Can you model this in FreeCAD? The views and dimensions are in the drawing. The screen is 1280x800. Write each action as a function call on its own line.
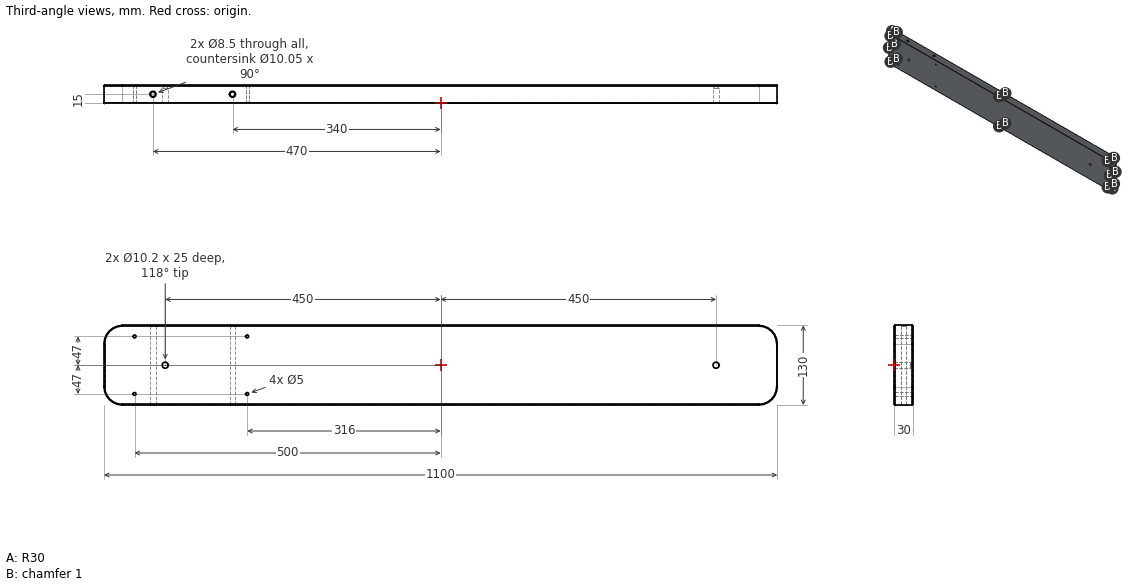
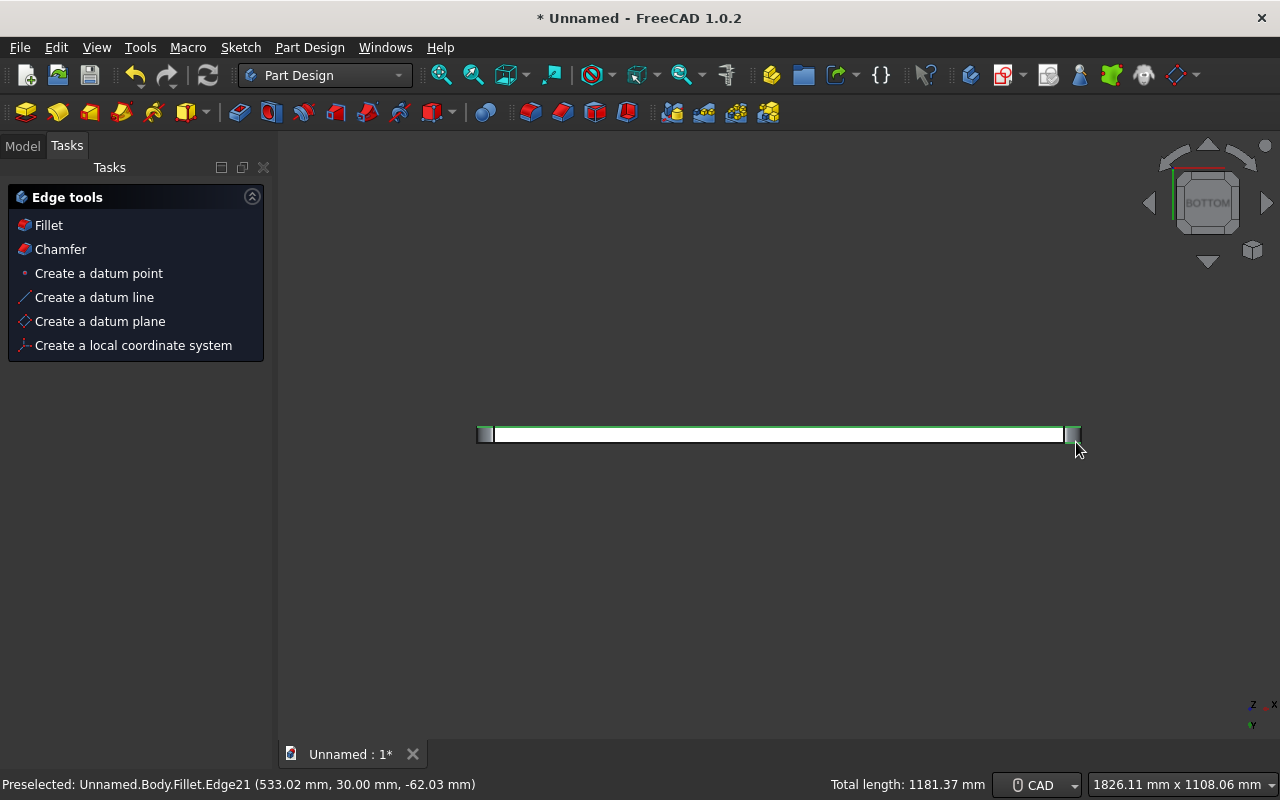
click(482, 442, ctrl)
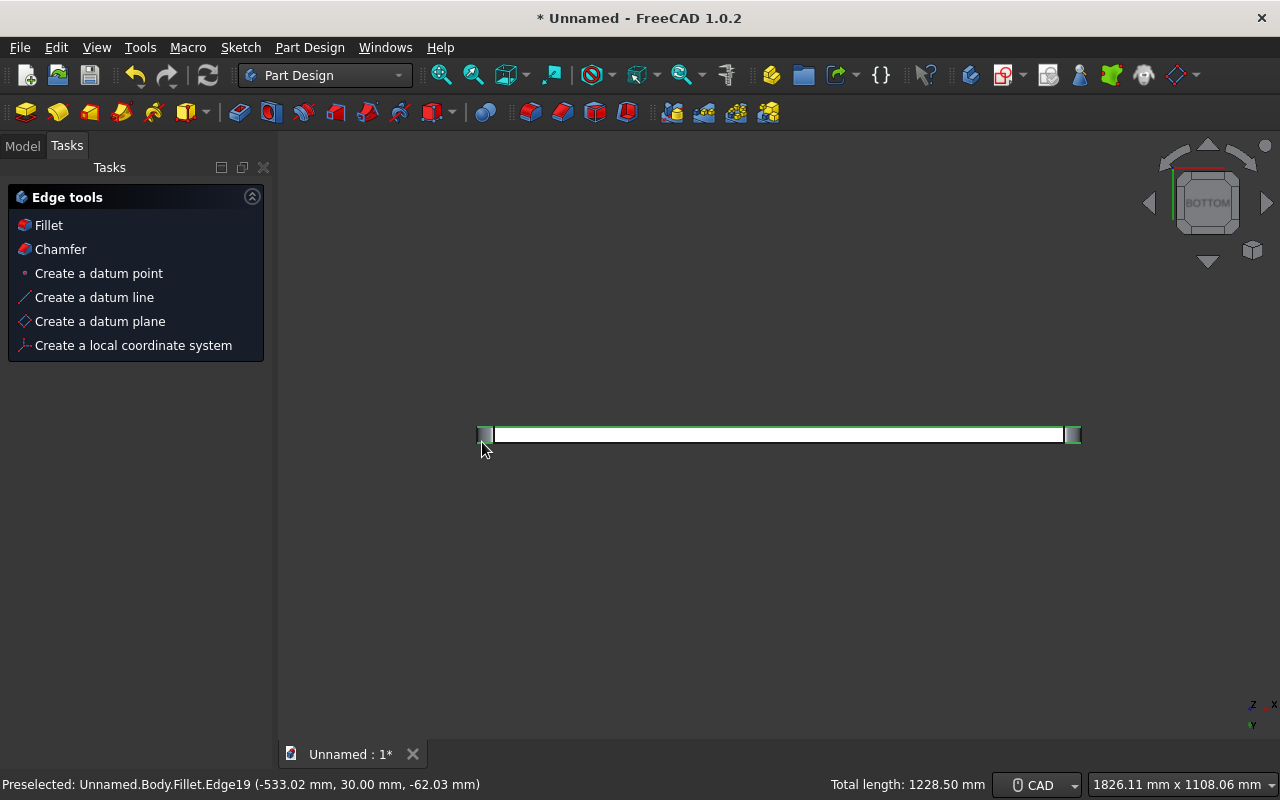
key(0)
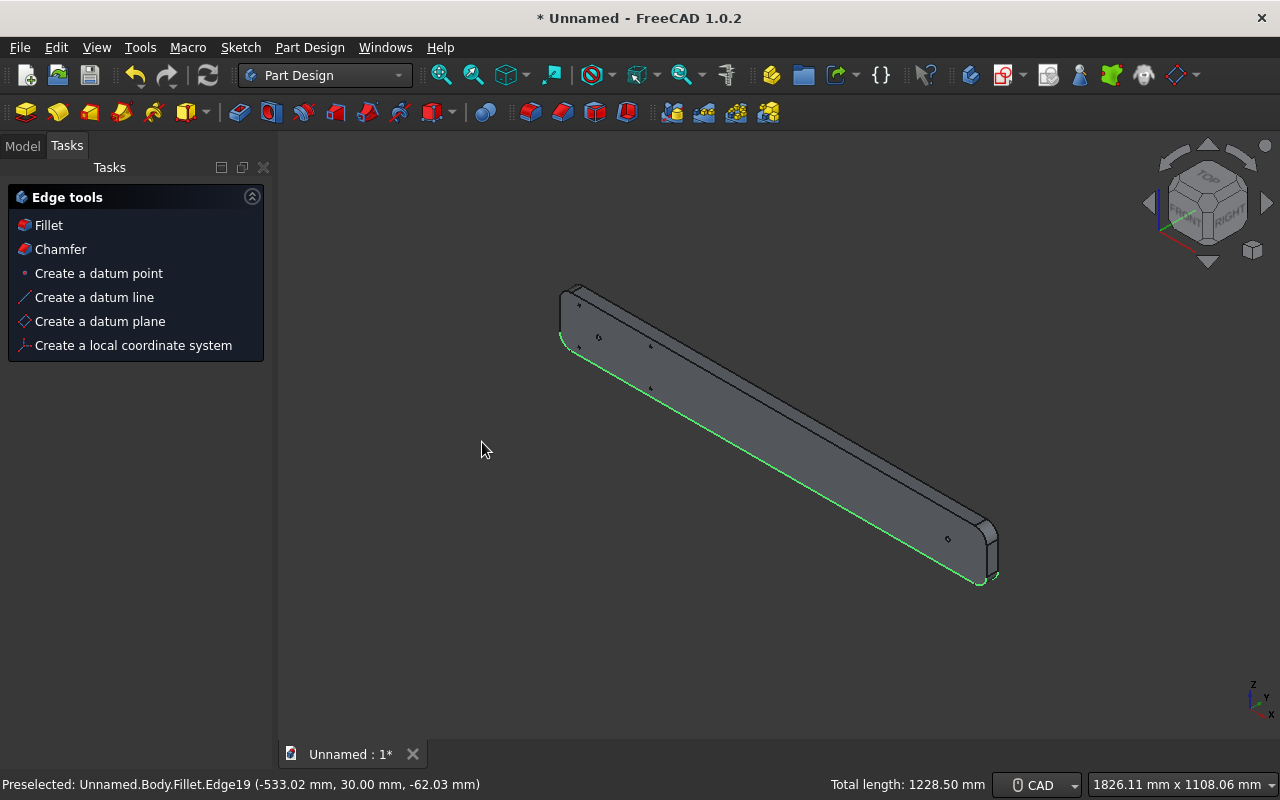
click(987, 561, ctrl)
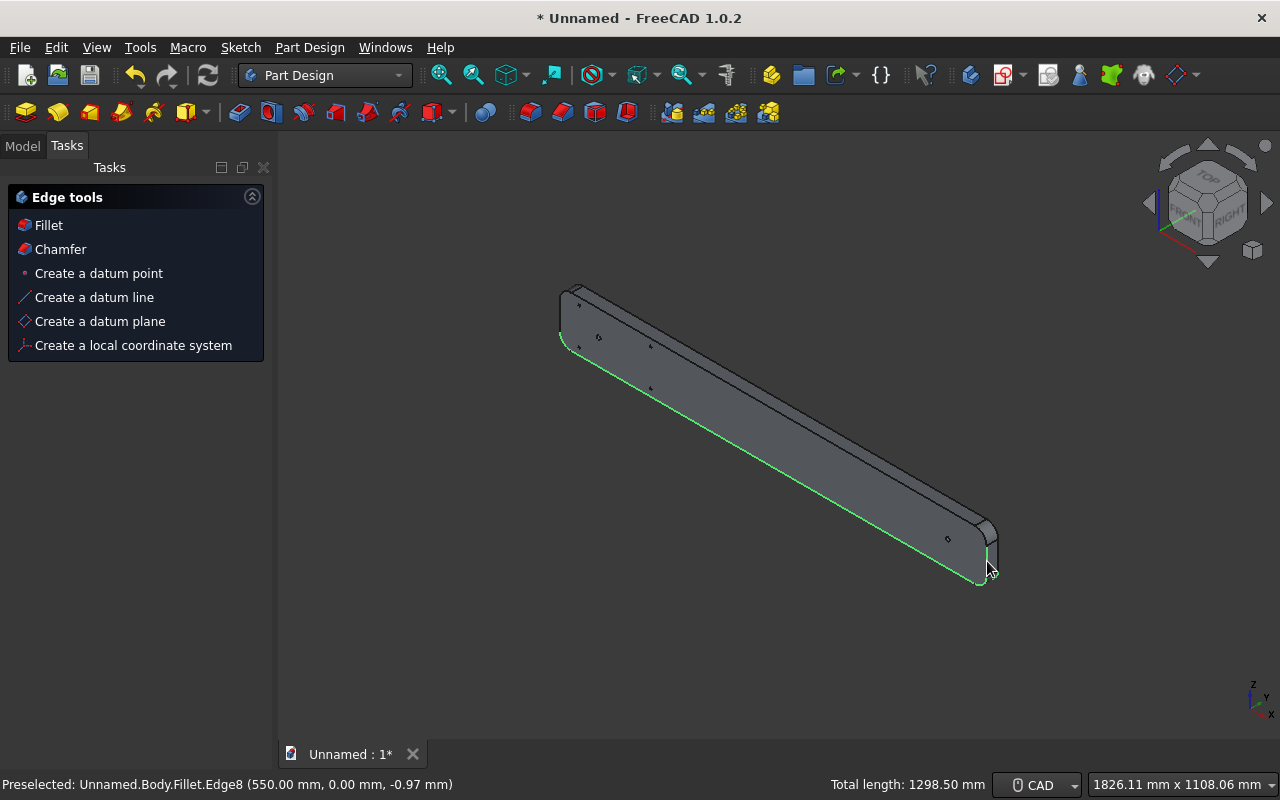
click(773, 408, ctrl)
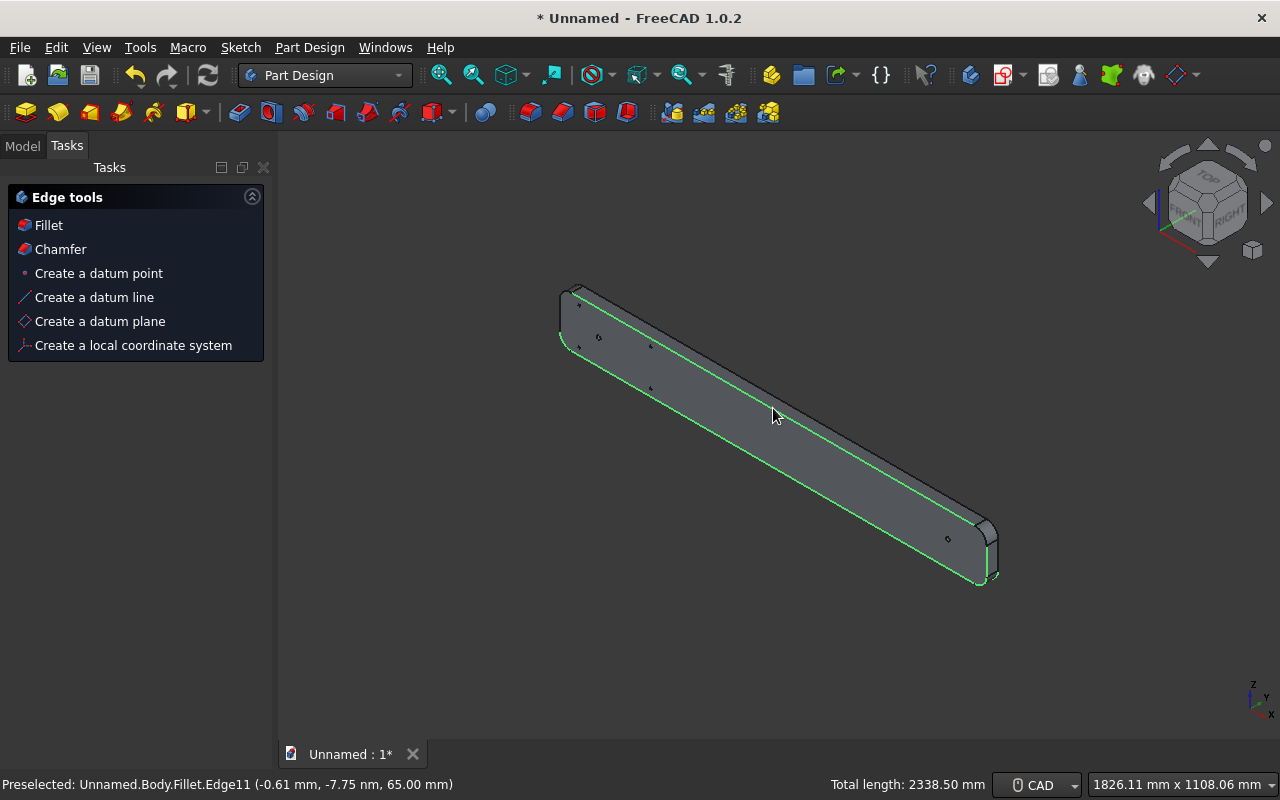
click(563, 291, ctrl)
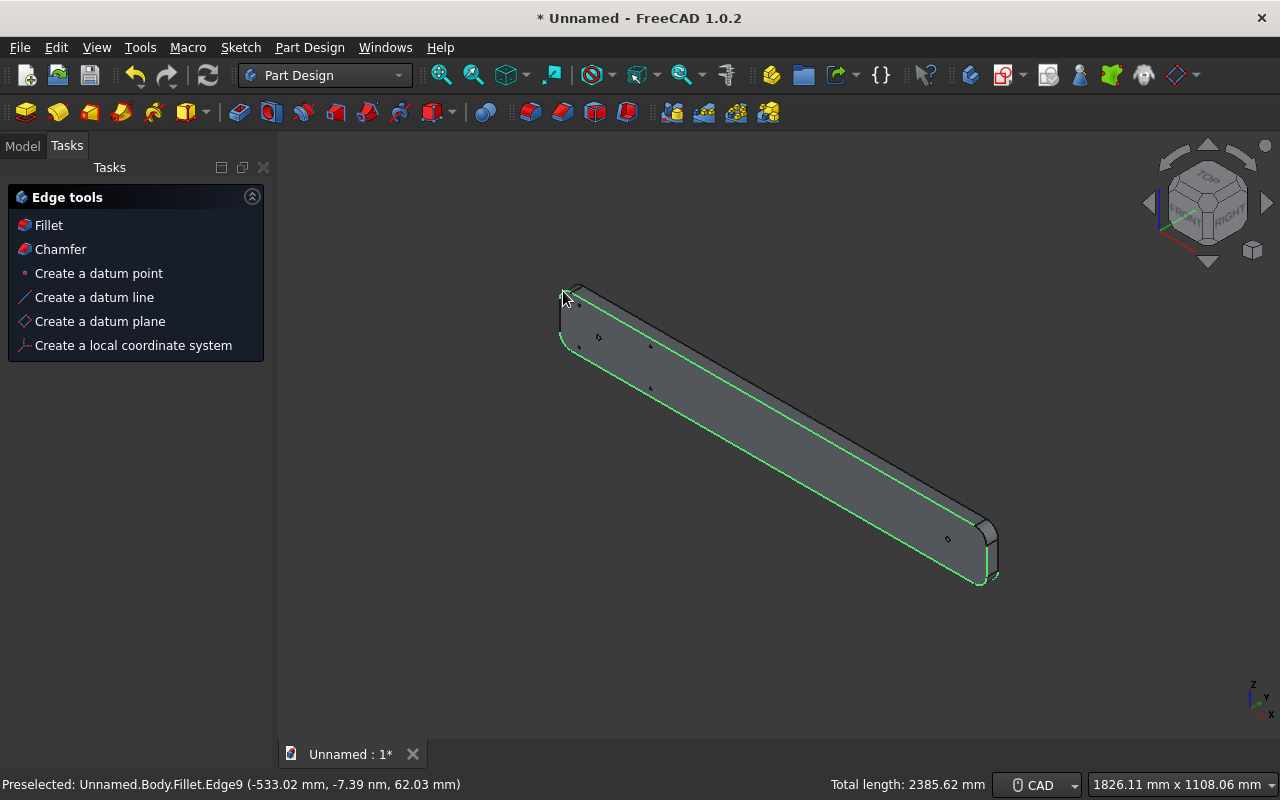
click(983, 533, ctrl)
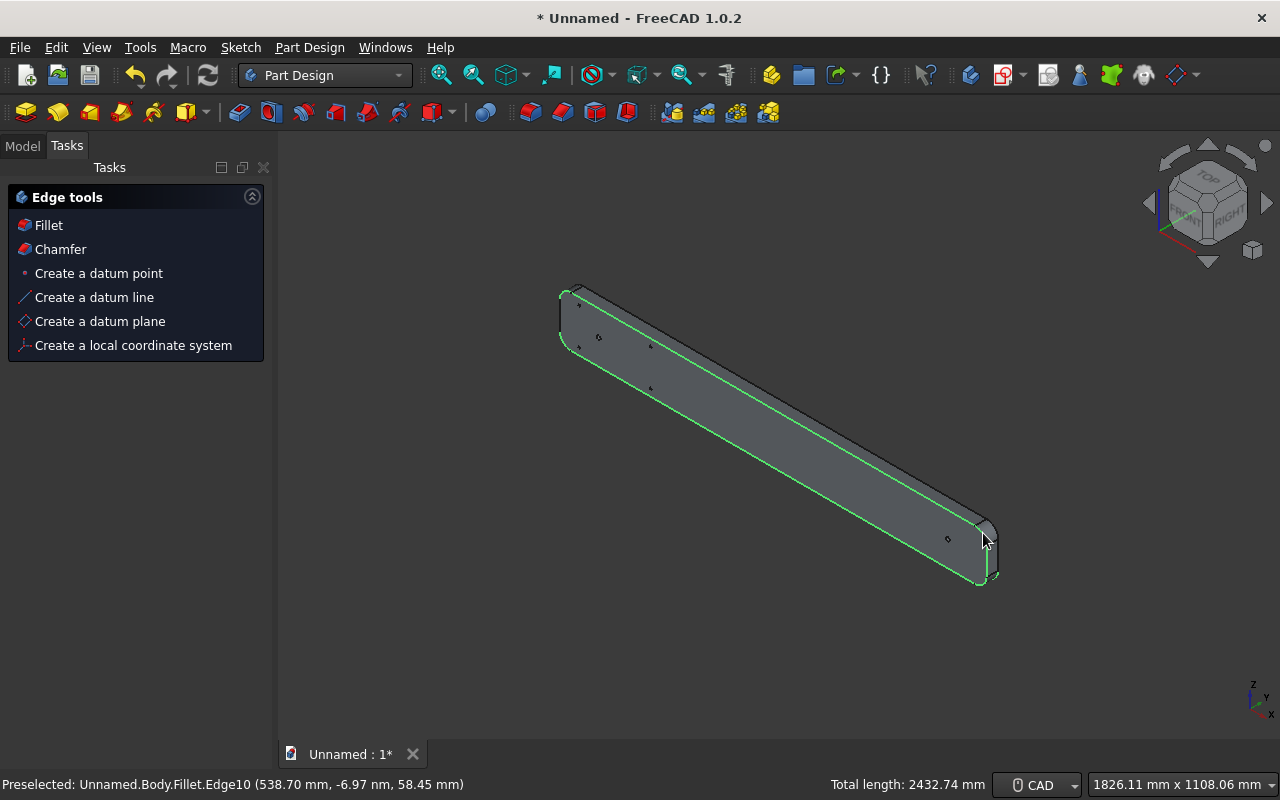
click(998, 534, ctrl)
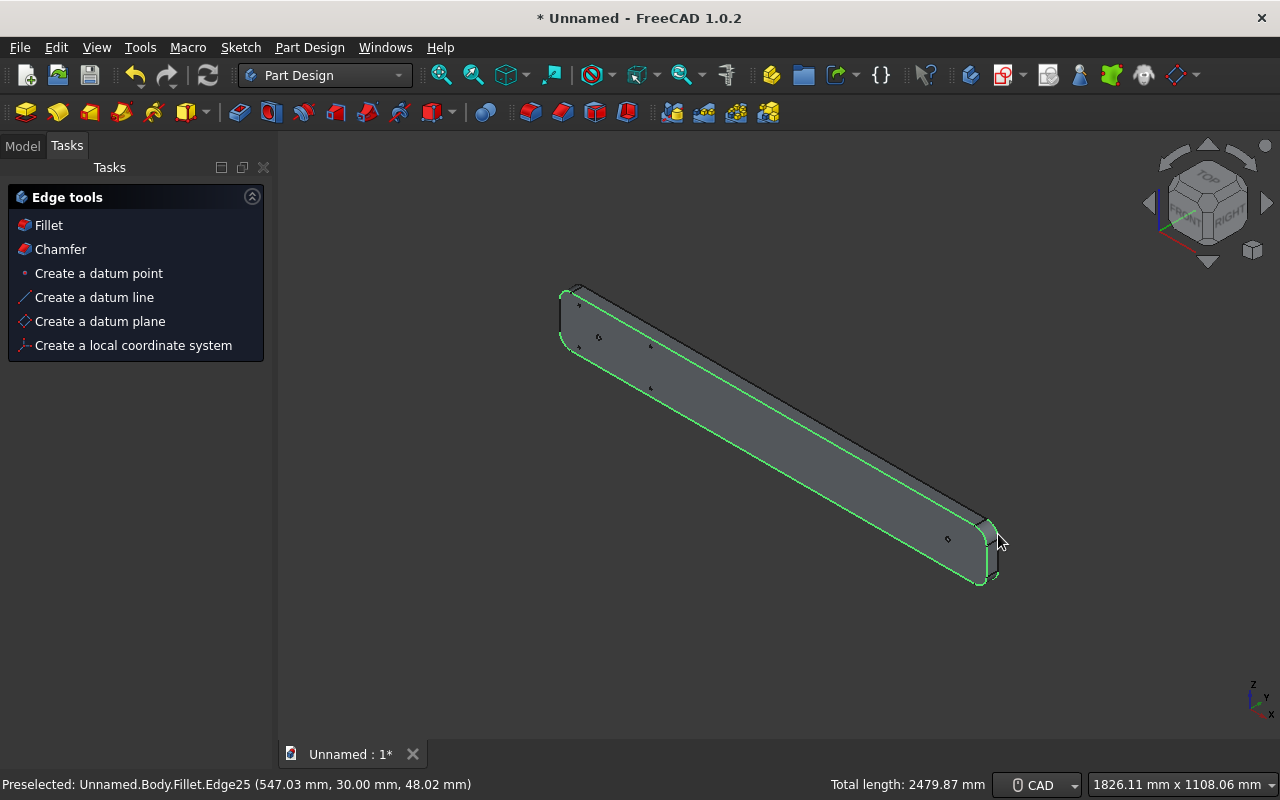
key(2)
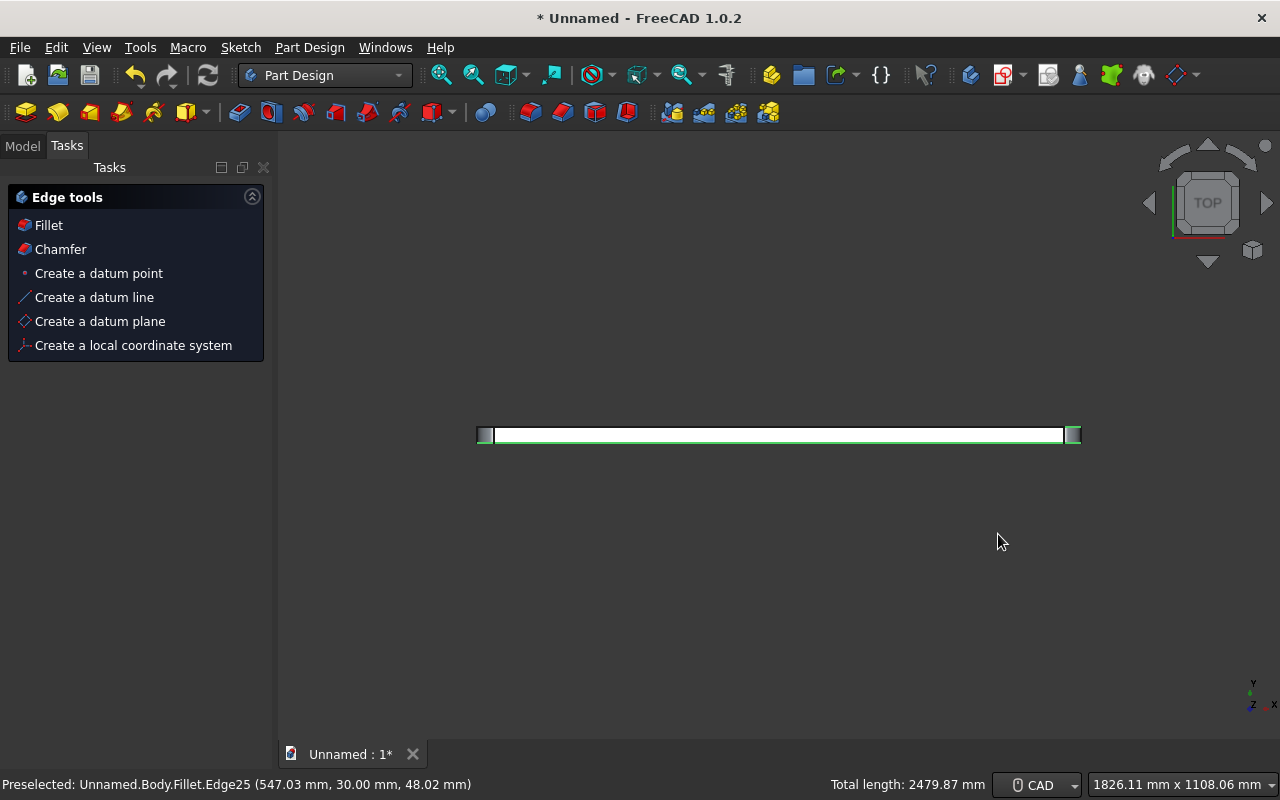
click(779, 426, ctrl)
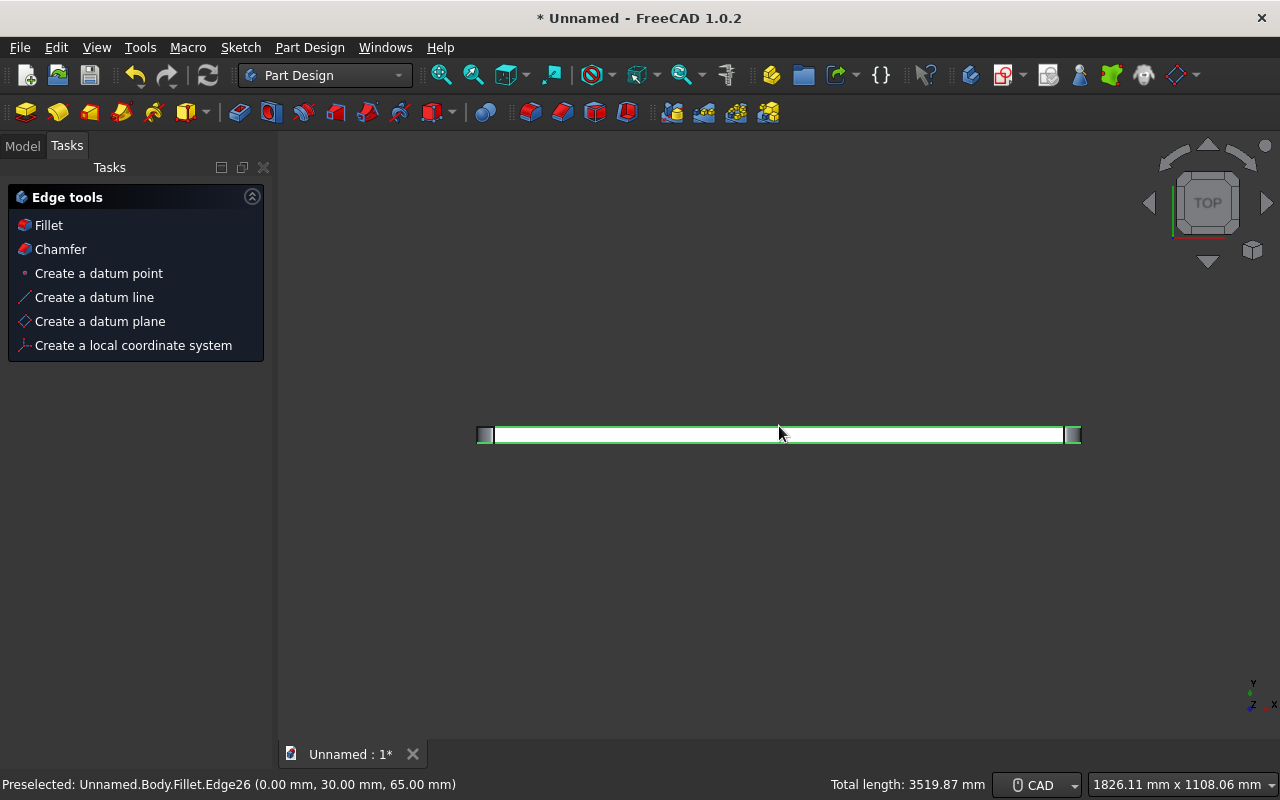
click(482, 426, ctrl)